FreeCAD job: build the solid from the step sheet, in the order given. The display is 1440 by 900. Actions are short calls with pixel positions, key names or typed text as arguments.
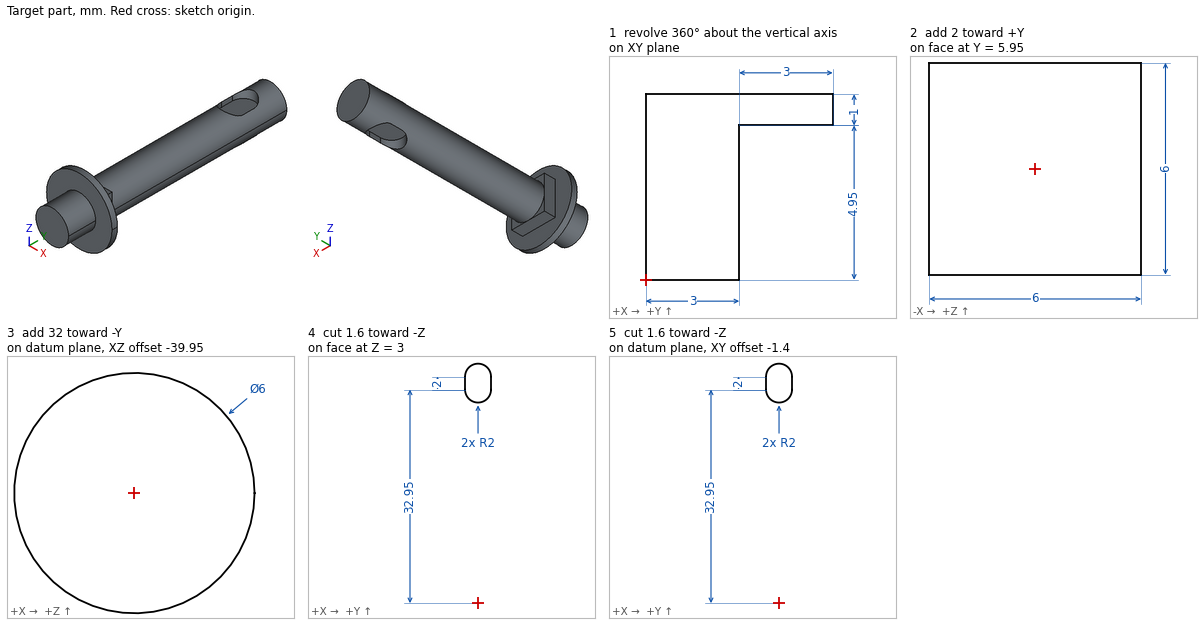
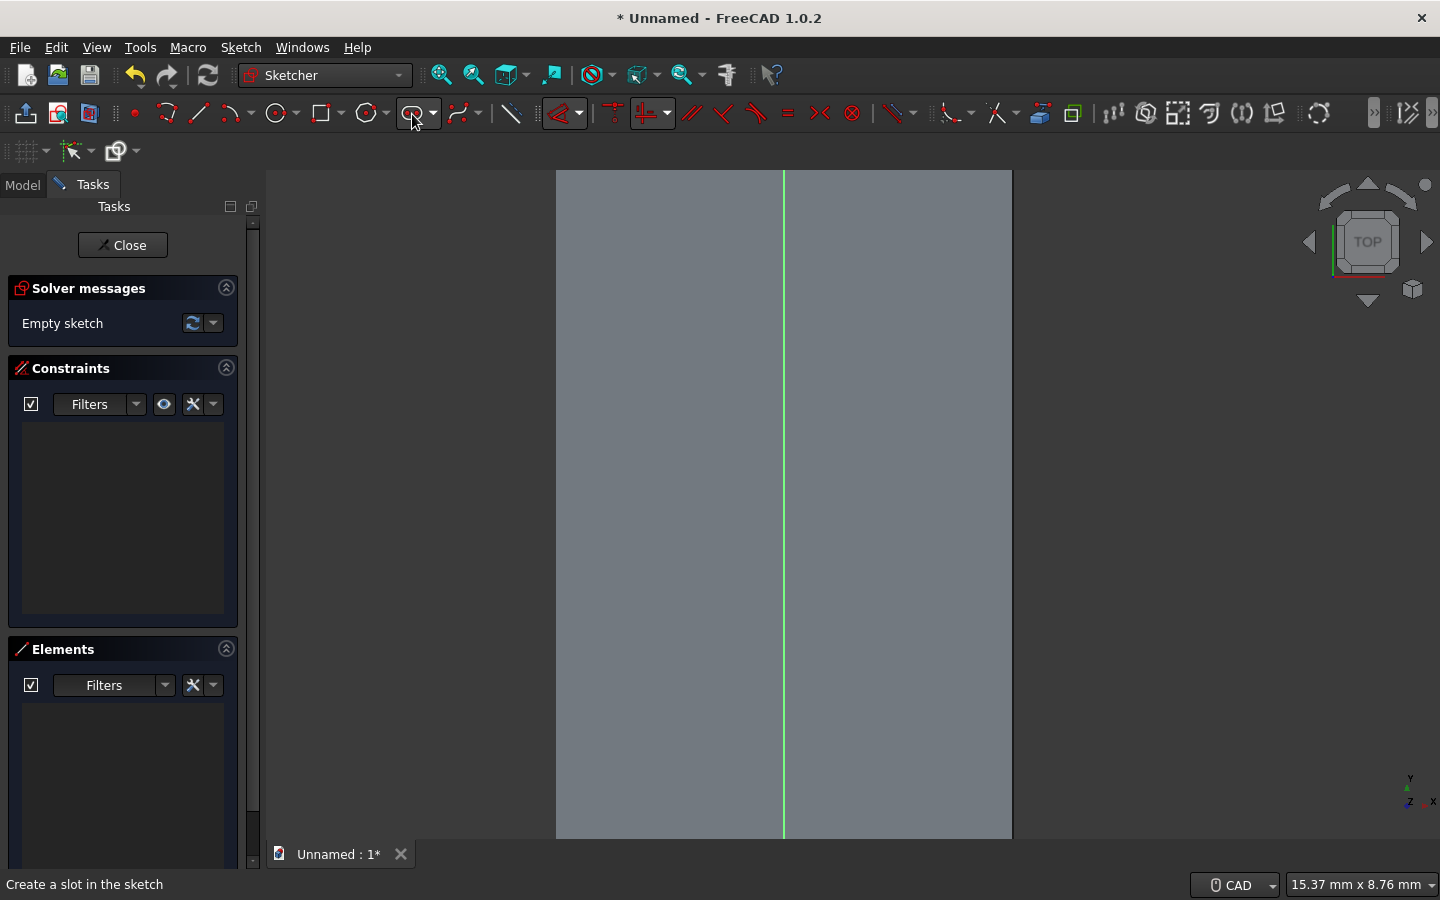
click(784, 579)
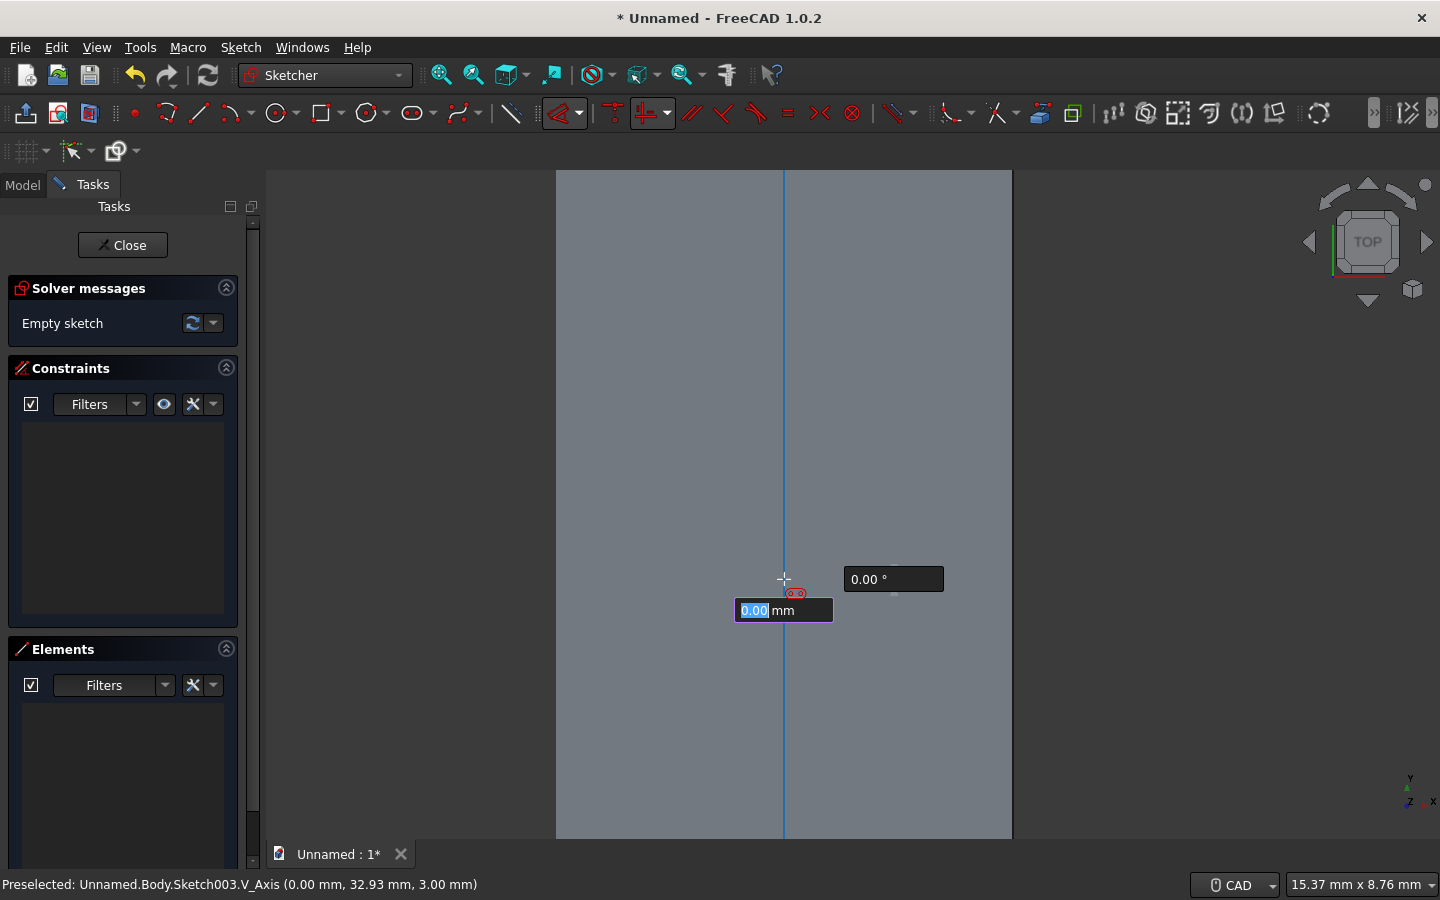
click(793, 426)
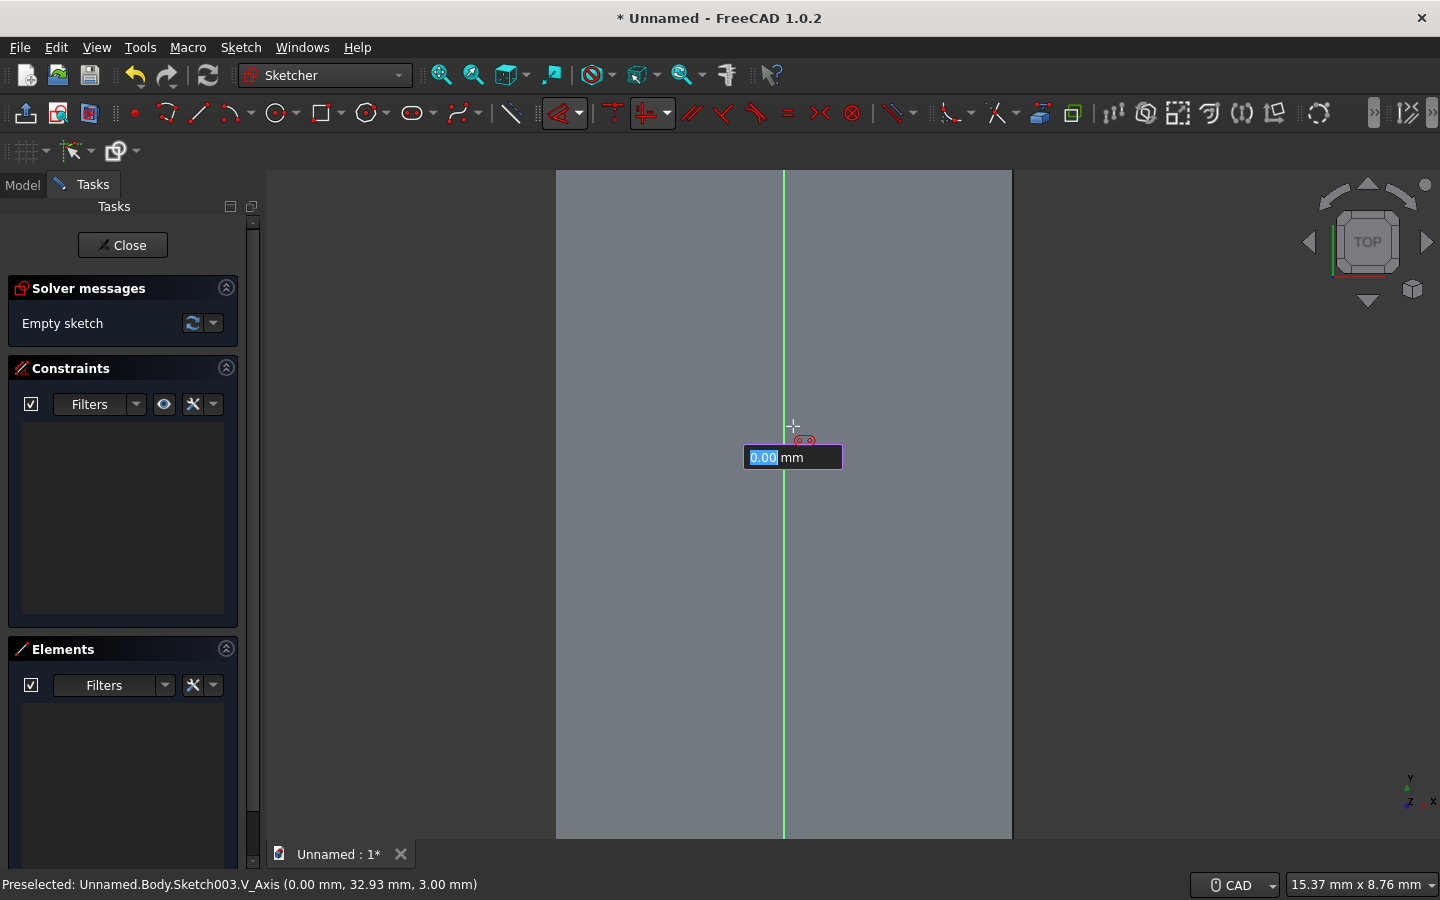
click(631, 502)
key(Escape)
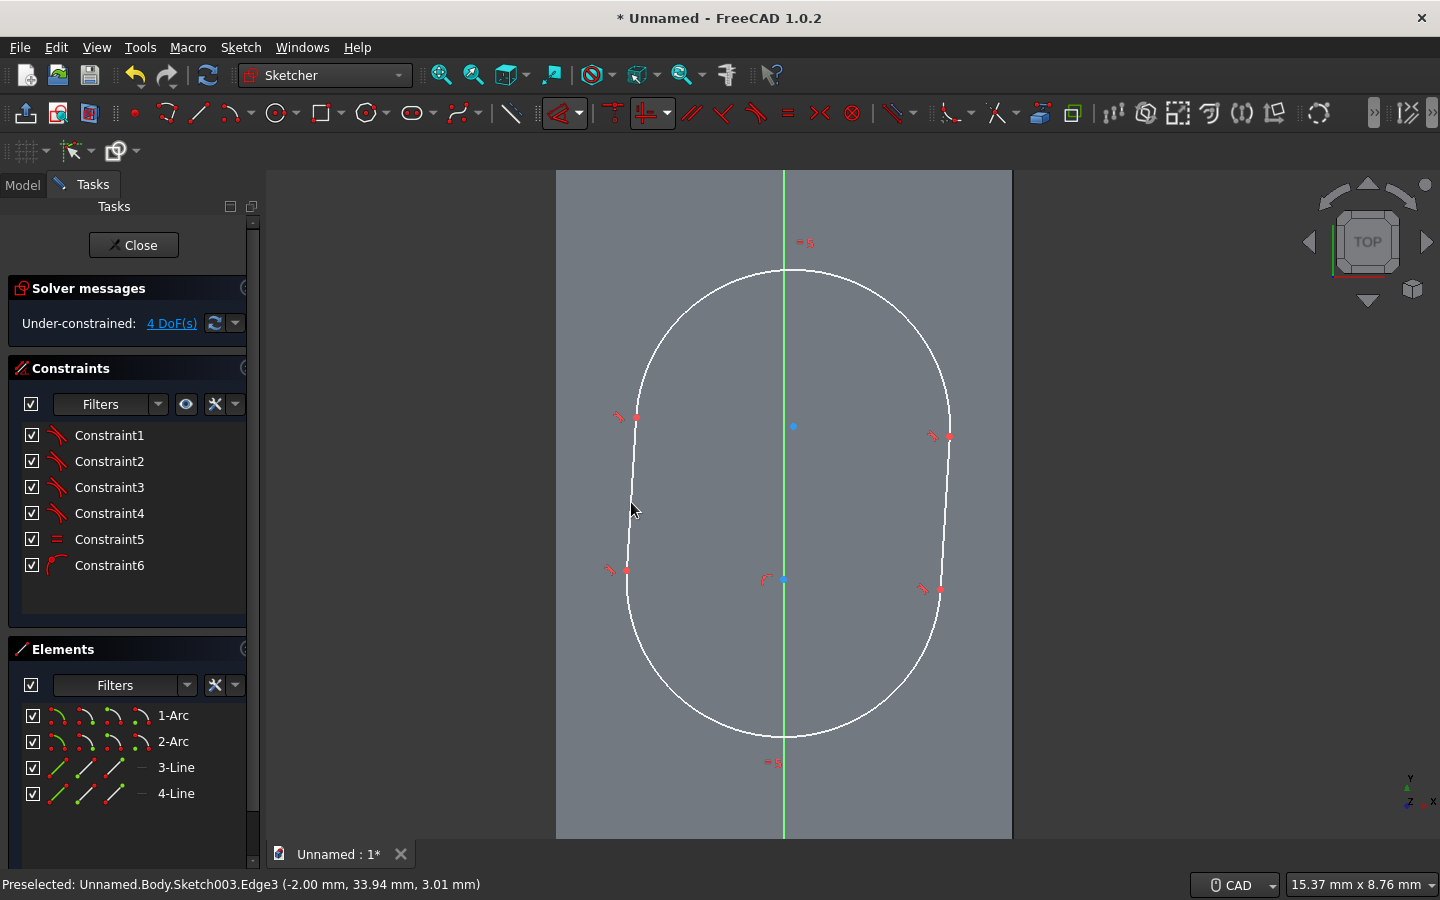
click(630, 525)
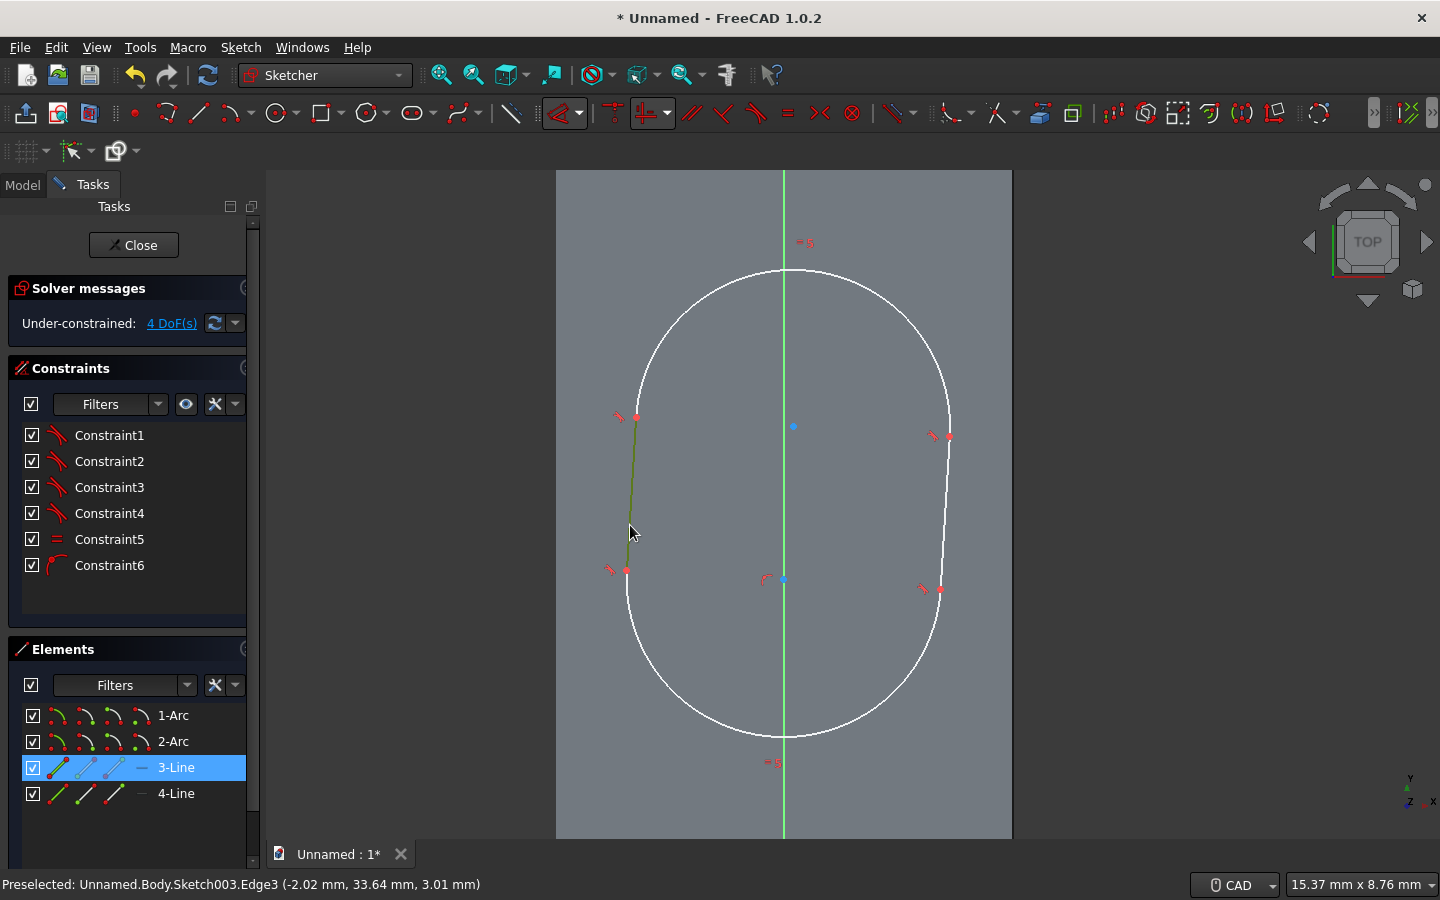
key(v)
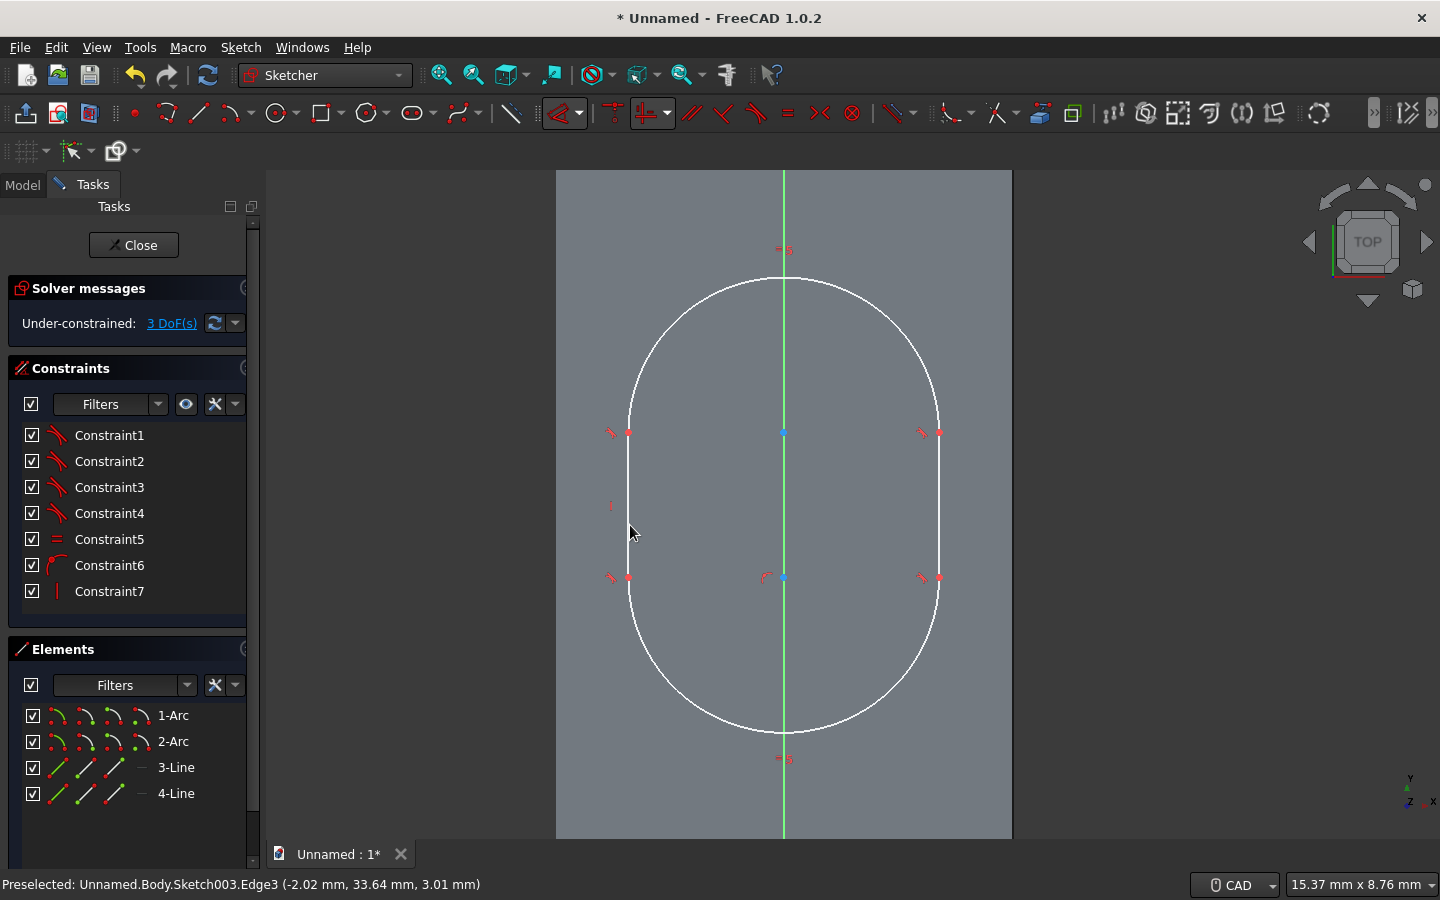
click(692, 703)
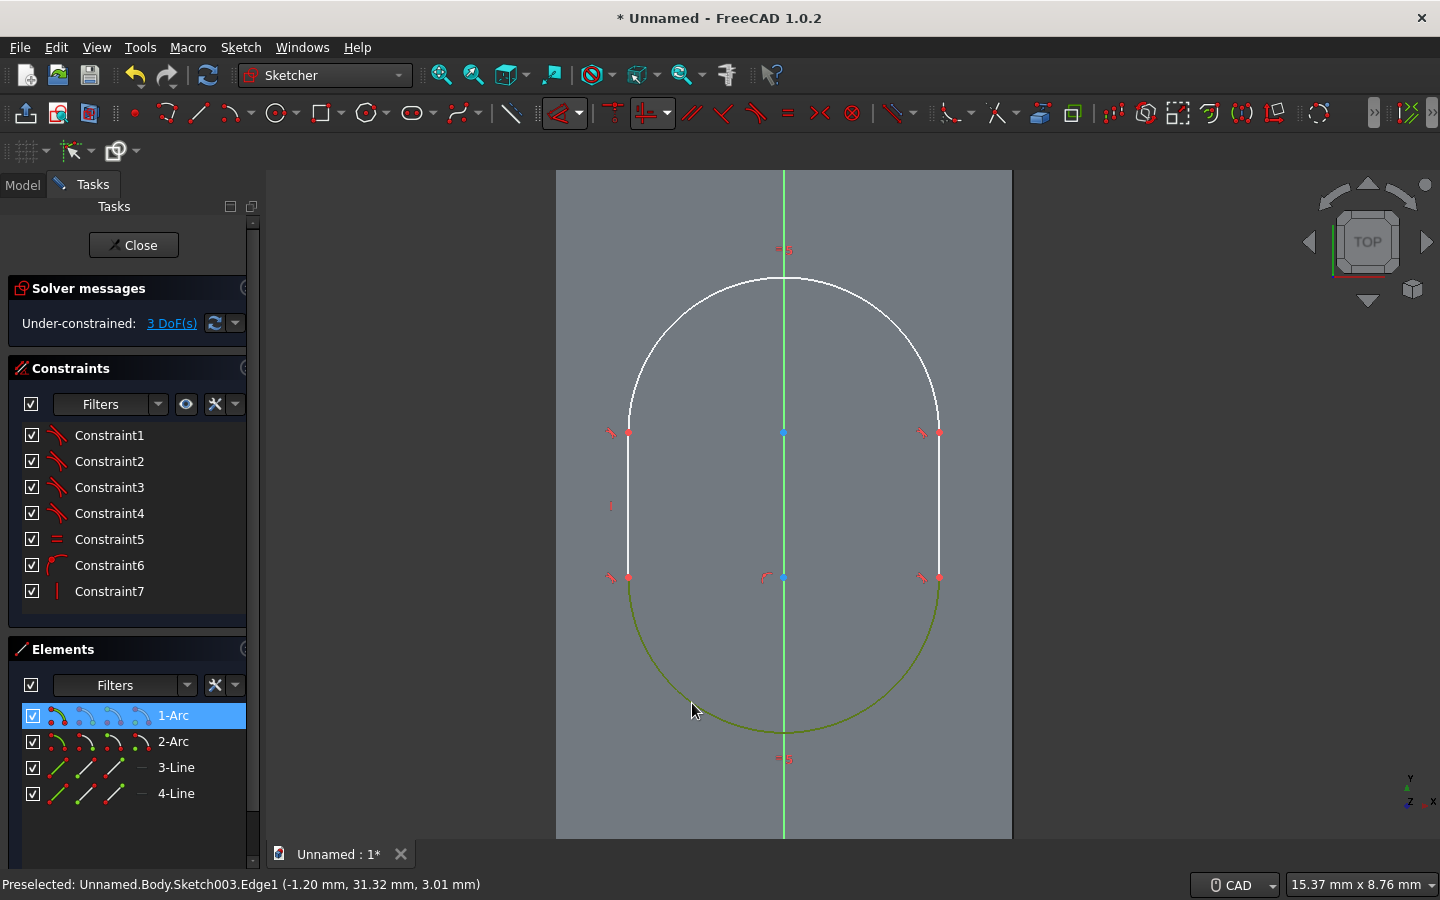
key(k)
key(r)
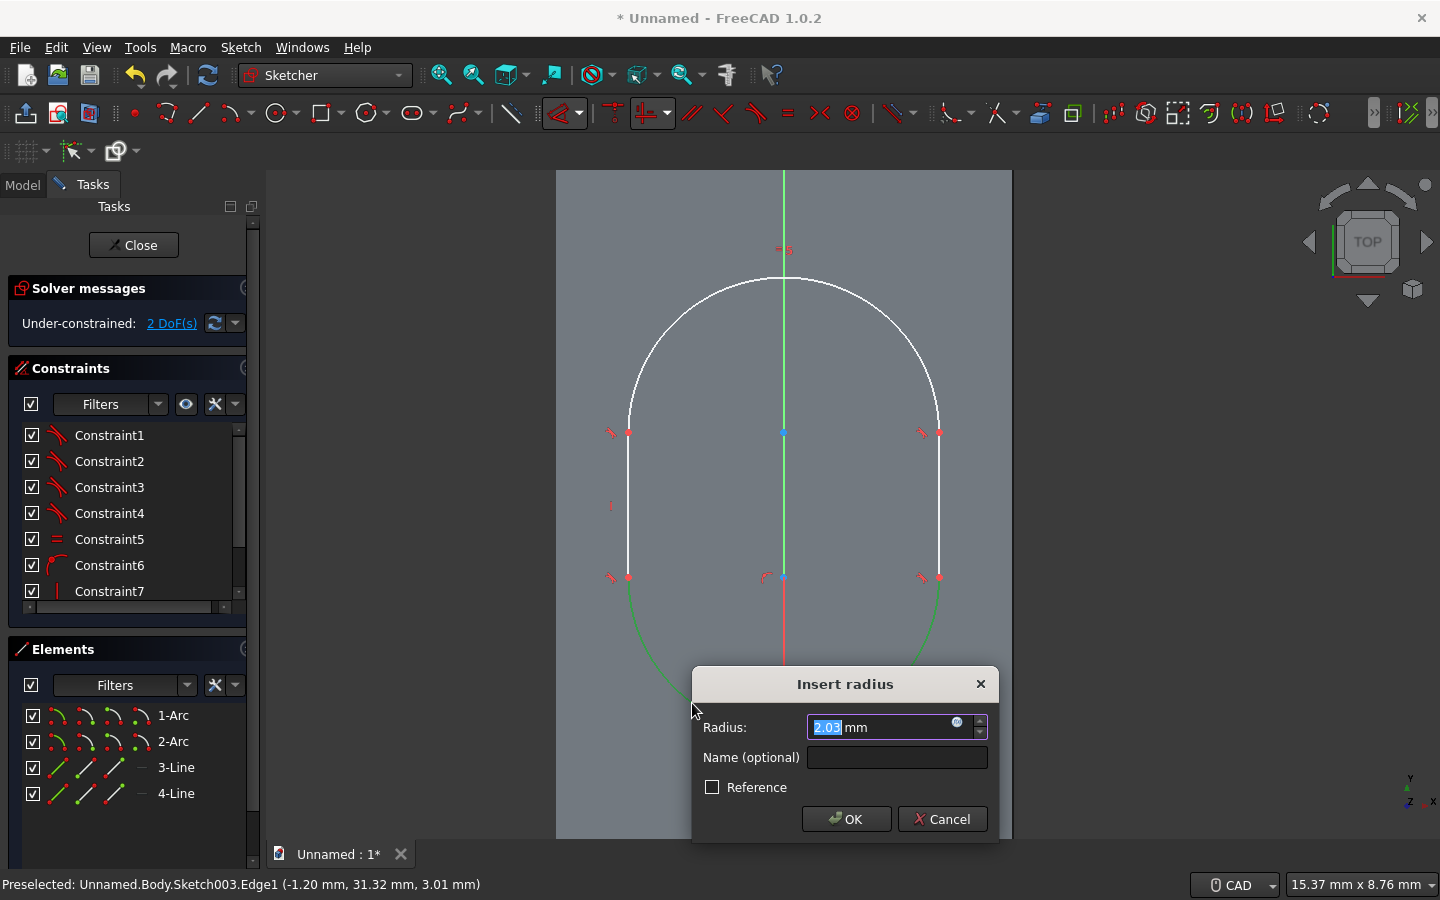
text(2)
key(Return)